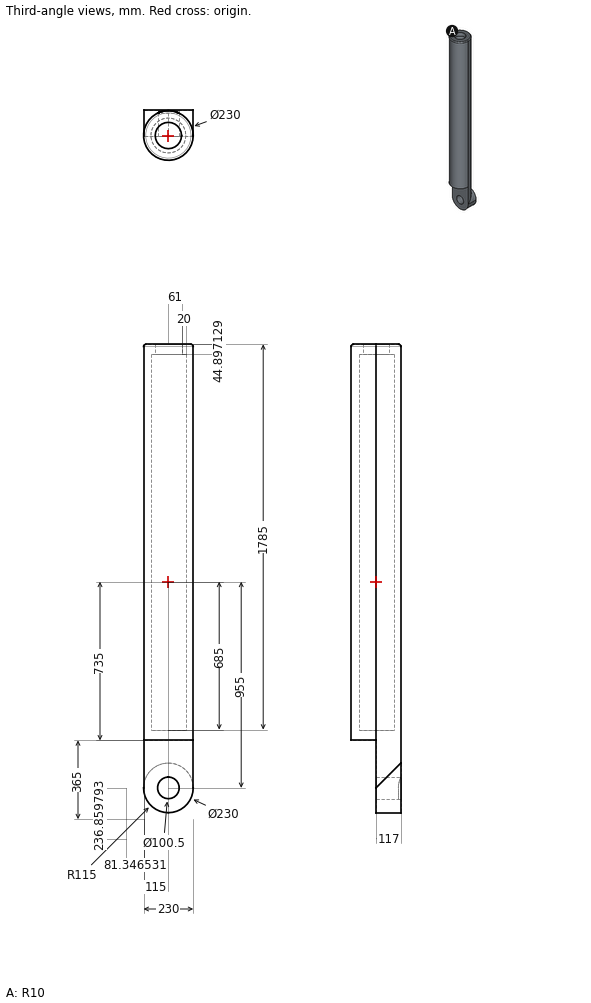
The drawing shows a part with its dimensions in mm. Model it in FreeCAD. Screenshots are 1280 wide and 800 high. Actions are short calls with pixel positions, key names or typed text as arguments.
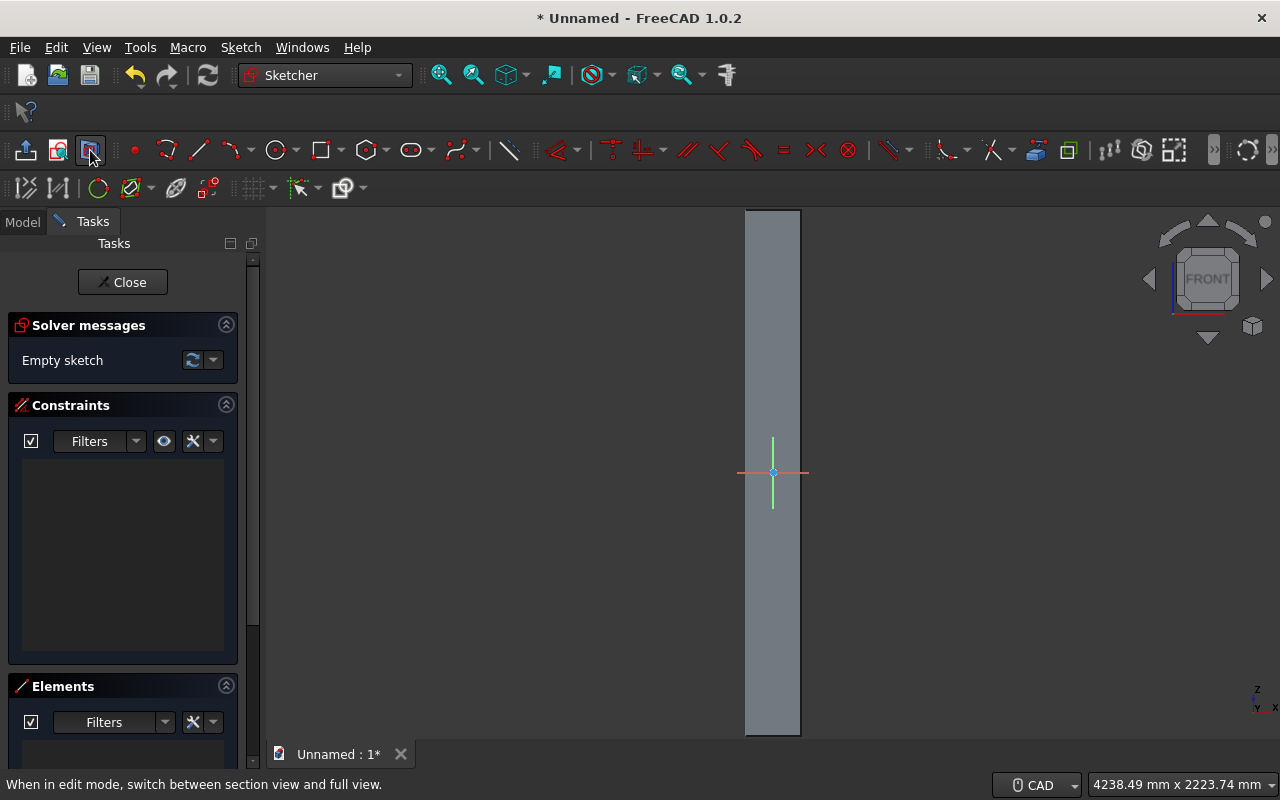
scroll(704, 473, down, 5)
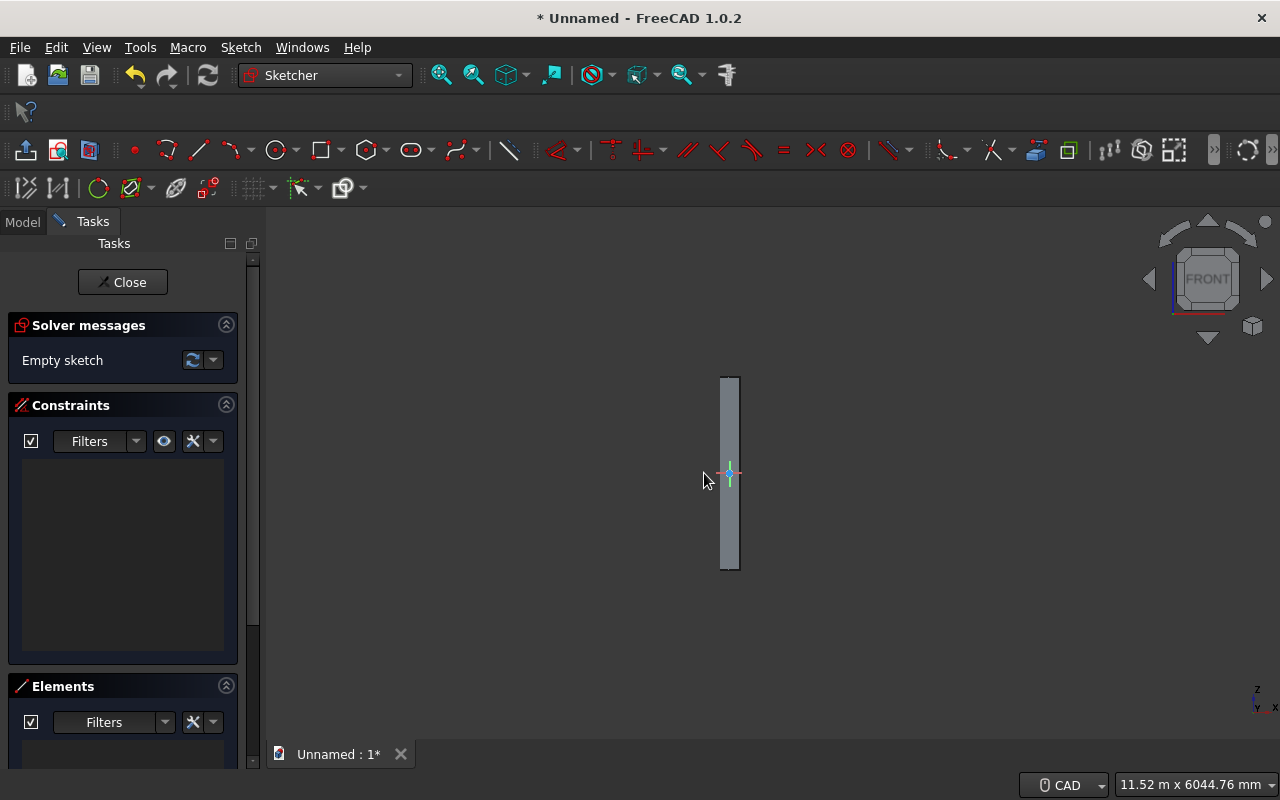
scroll(731, 562, up, 15)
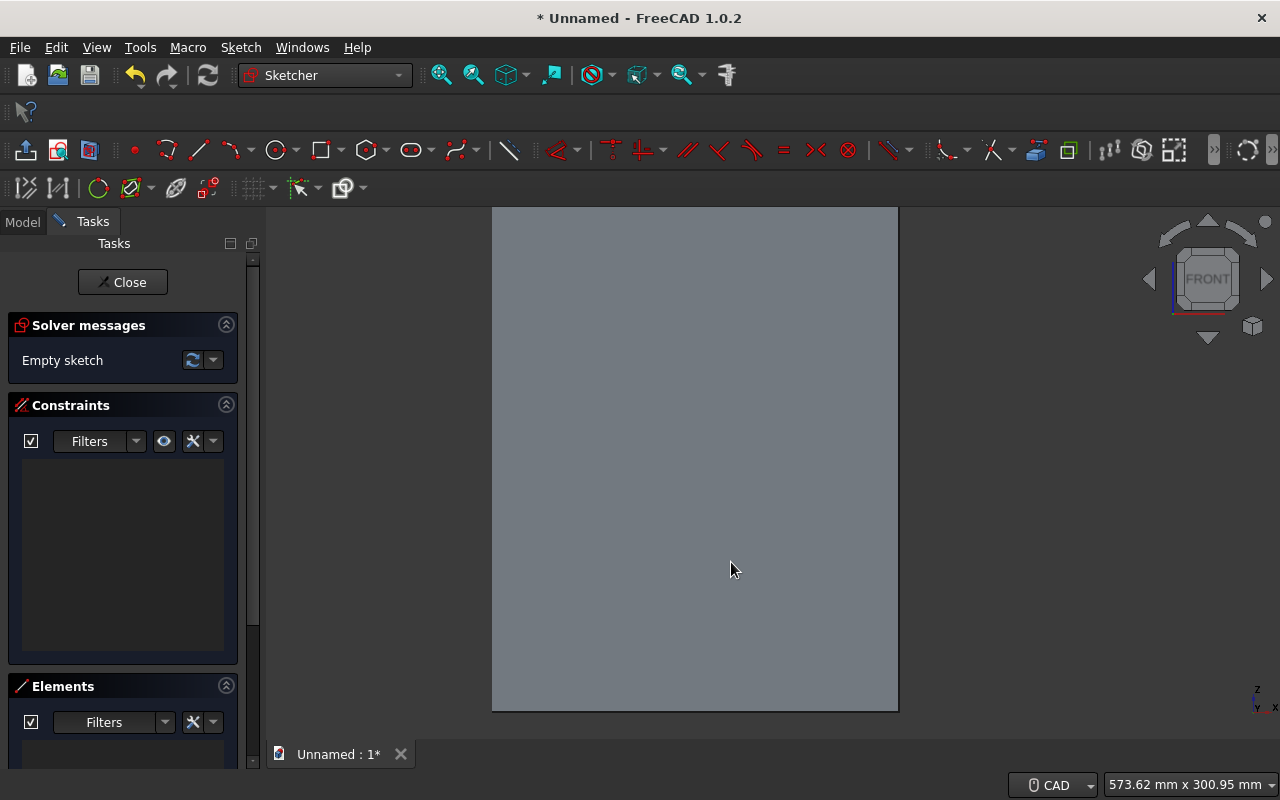
scroll(684, 436, up, 3)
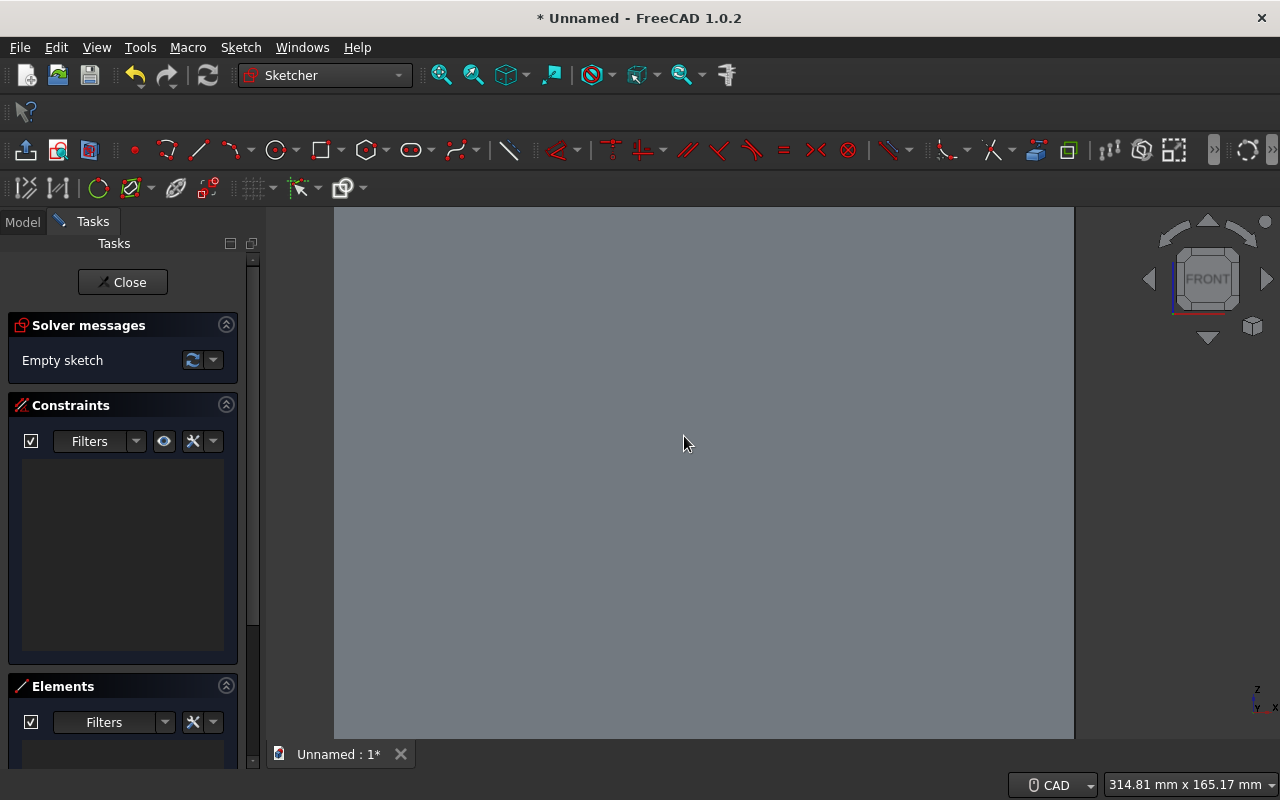
click(276, 150)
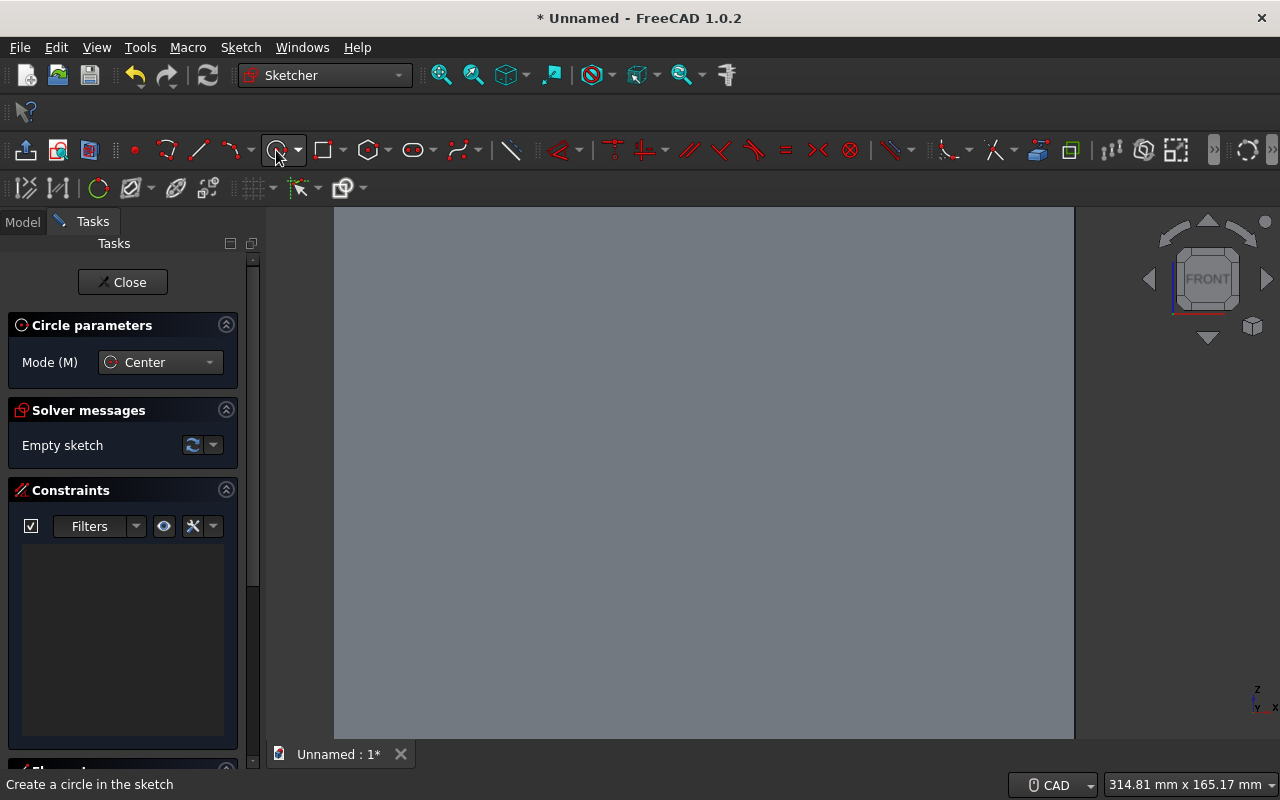
click(704, 472)
click(819, 358)
key(Escape)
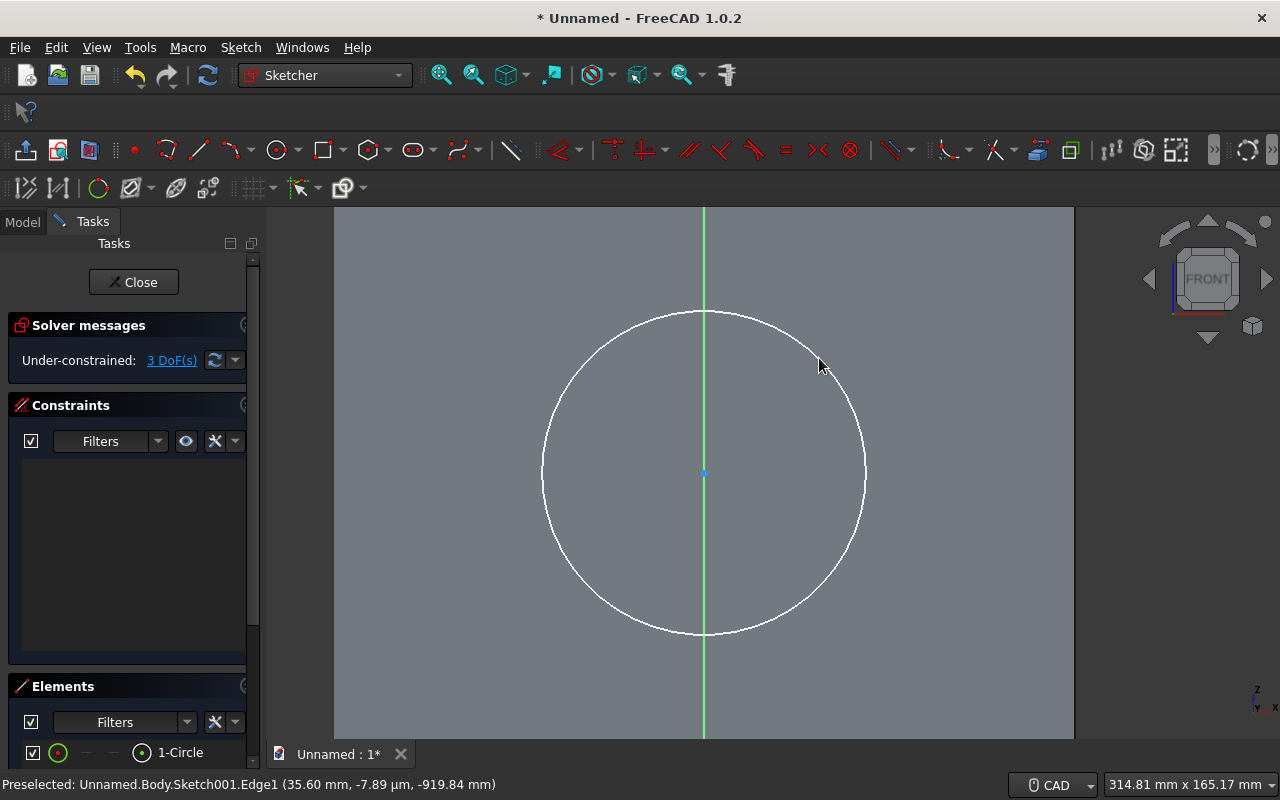
click(704, 473)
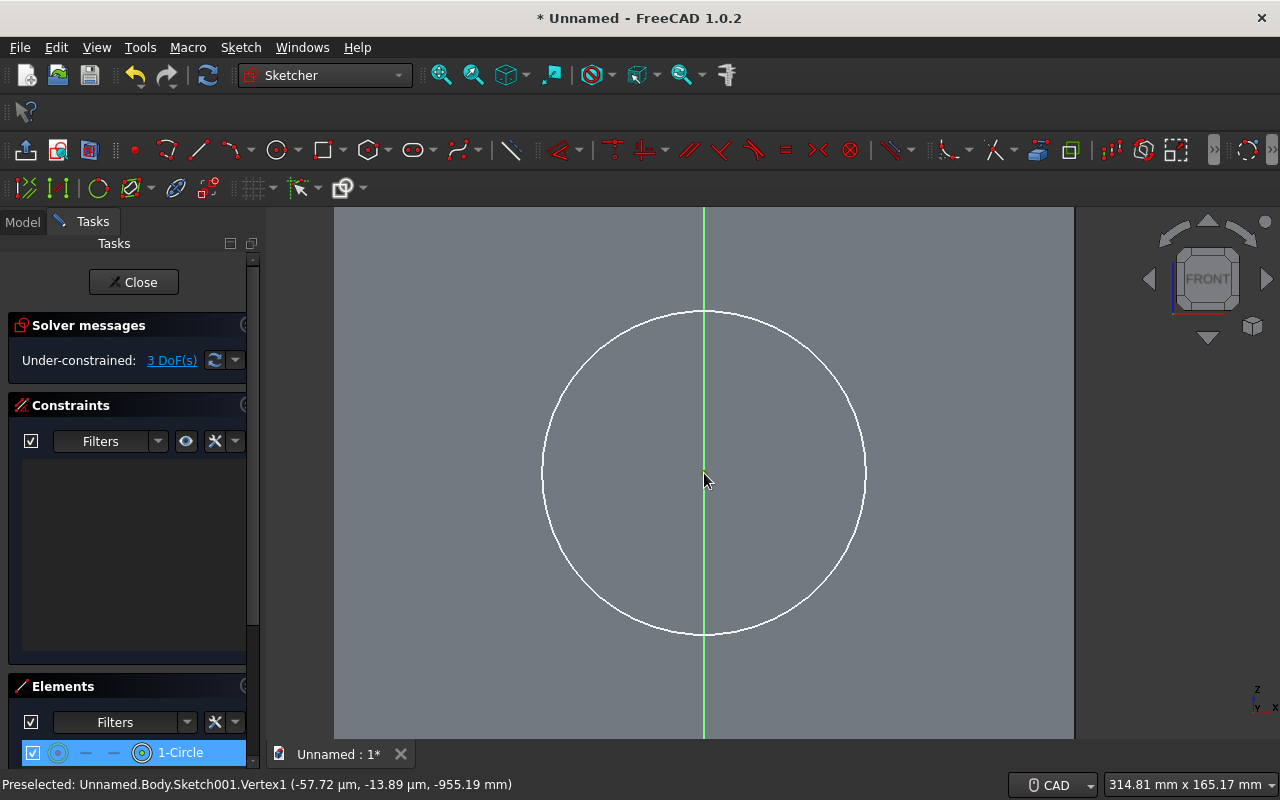
click(704, 677)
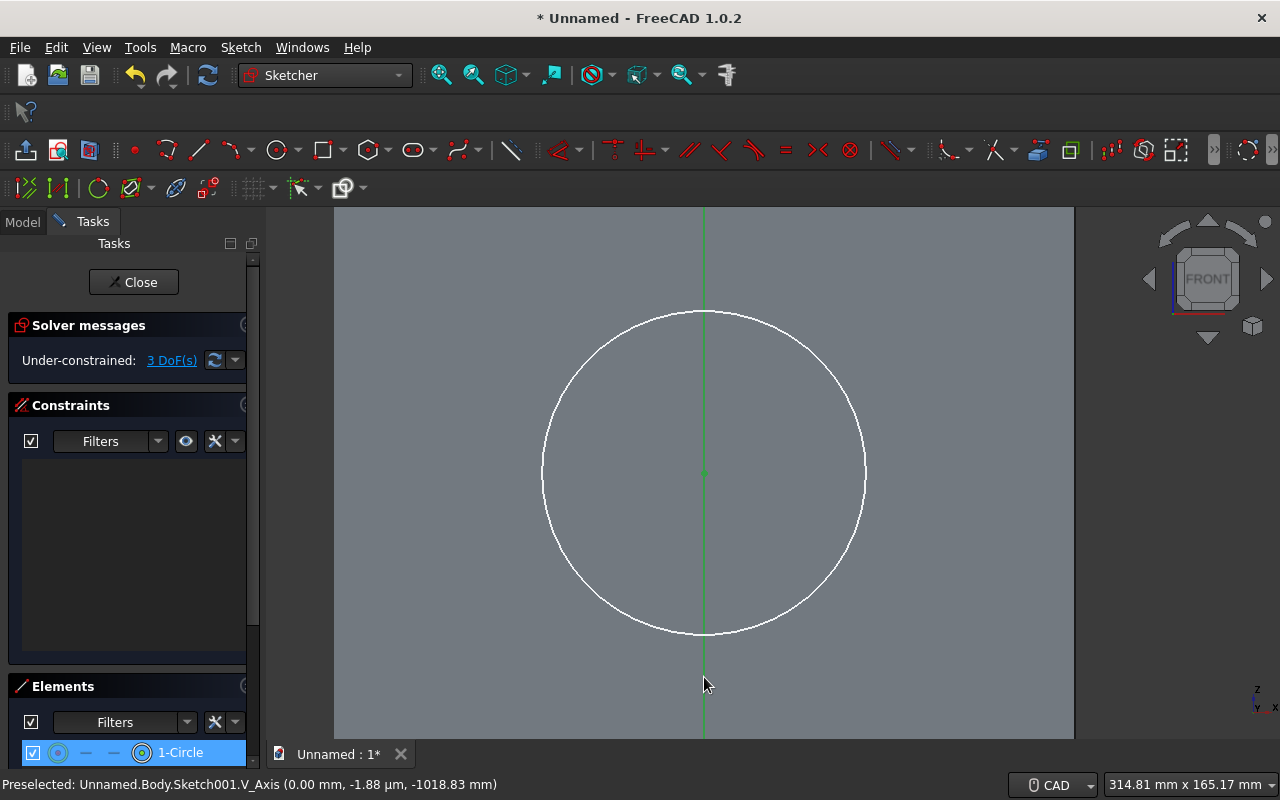
click(614, 150)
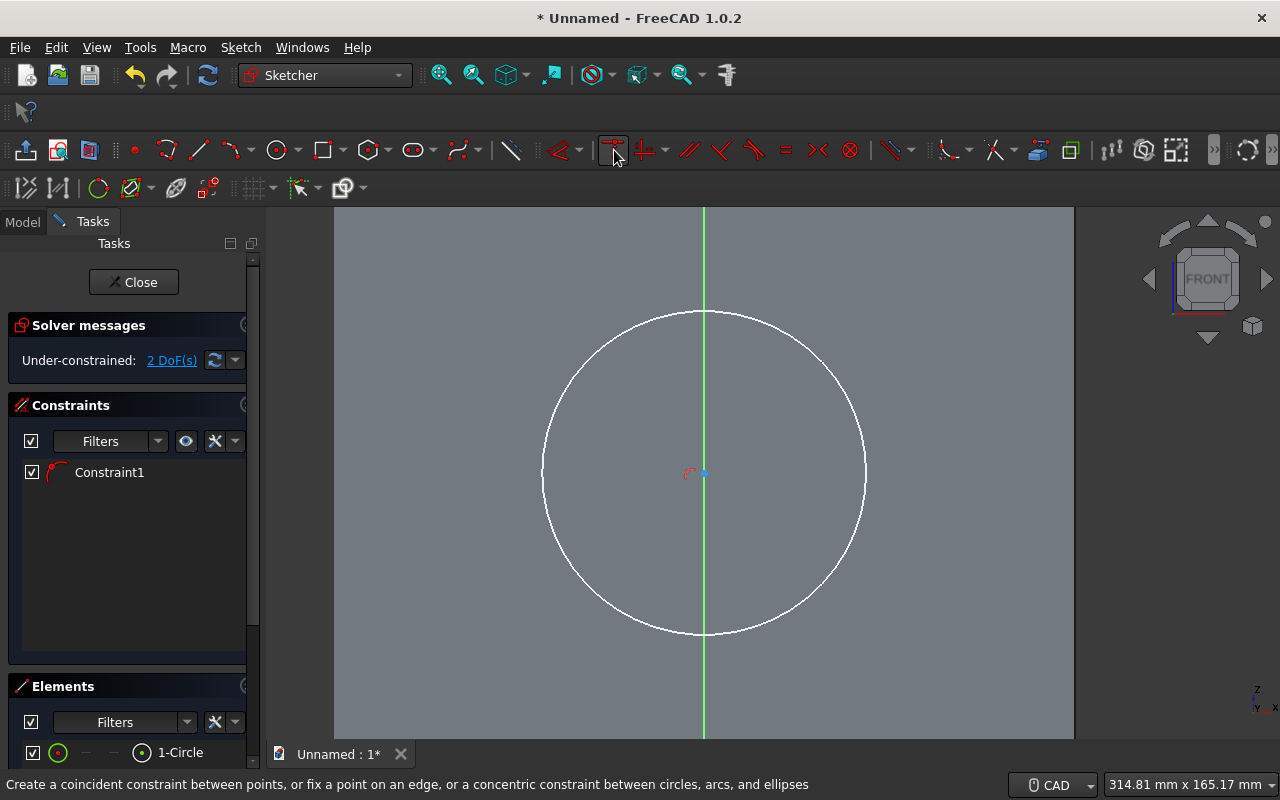
click(558, 150)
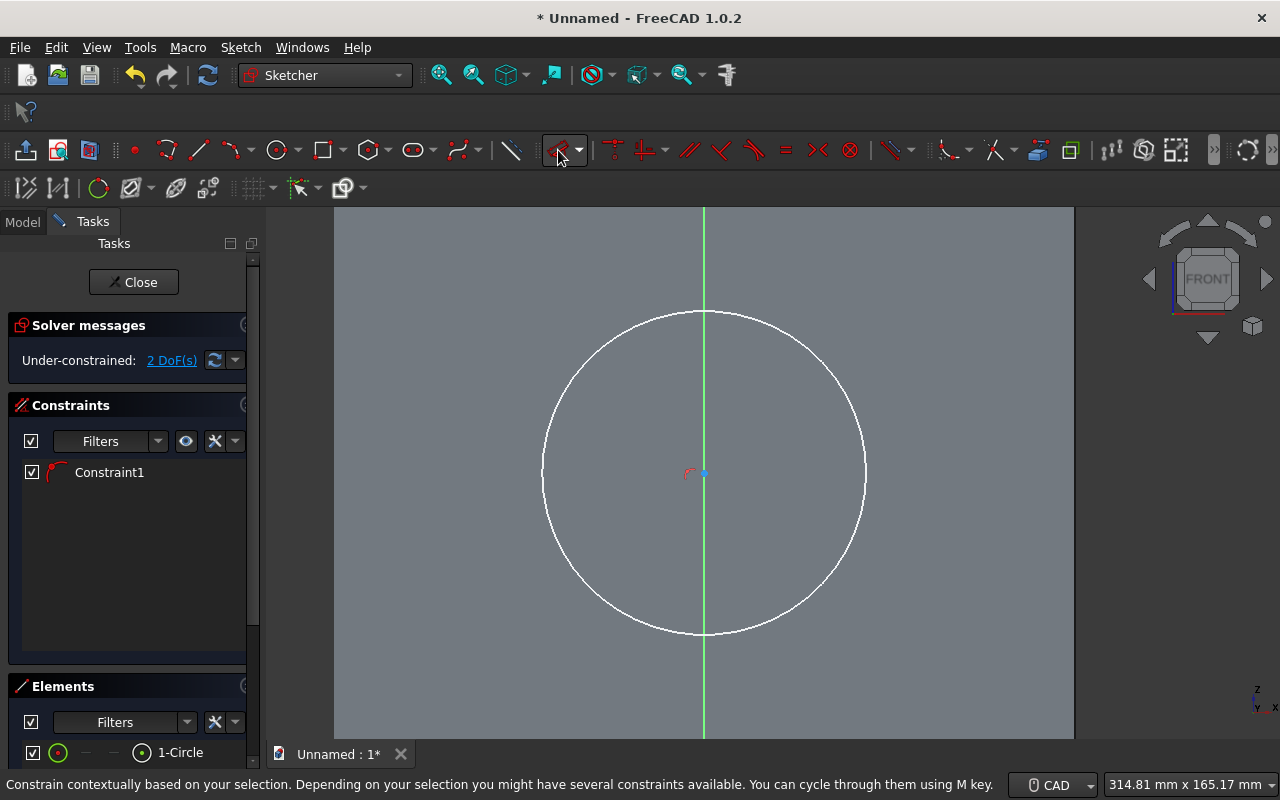
click(818, 358)
click(841, 335)